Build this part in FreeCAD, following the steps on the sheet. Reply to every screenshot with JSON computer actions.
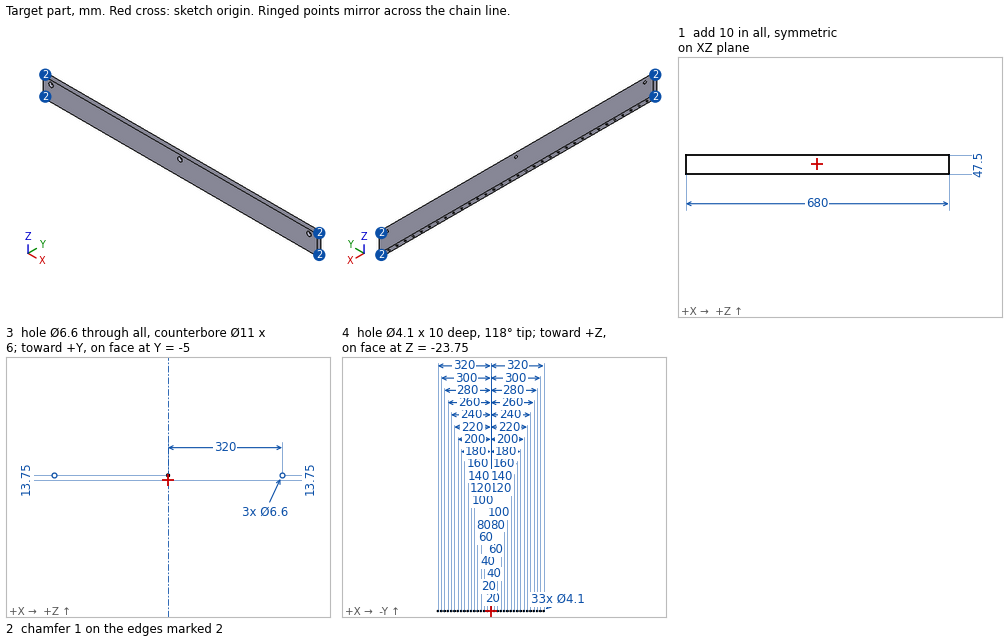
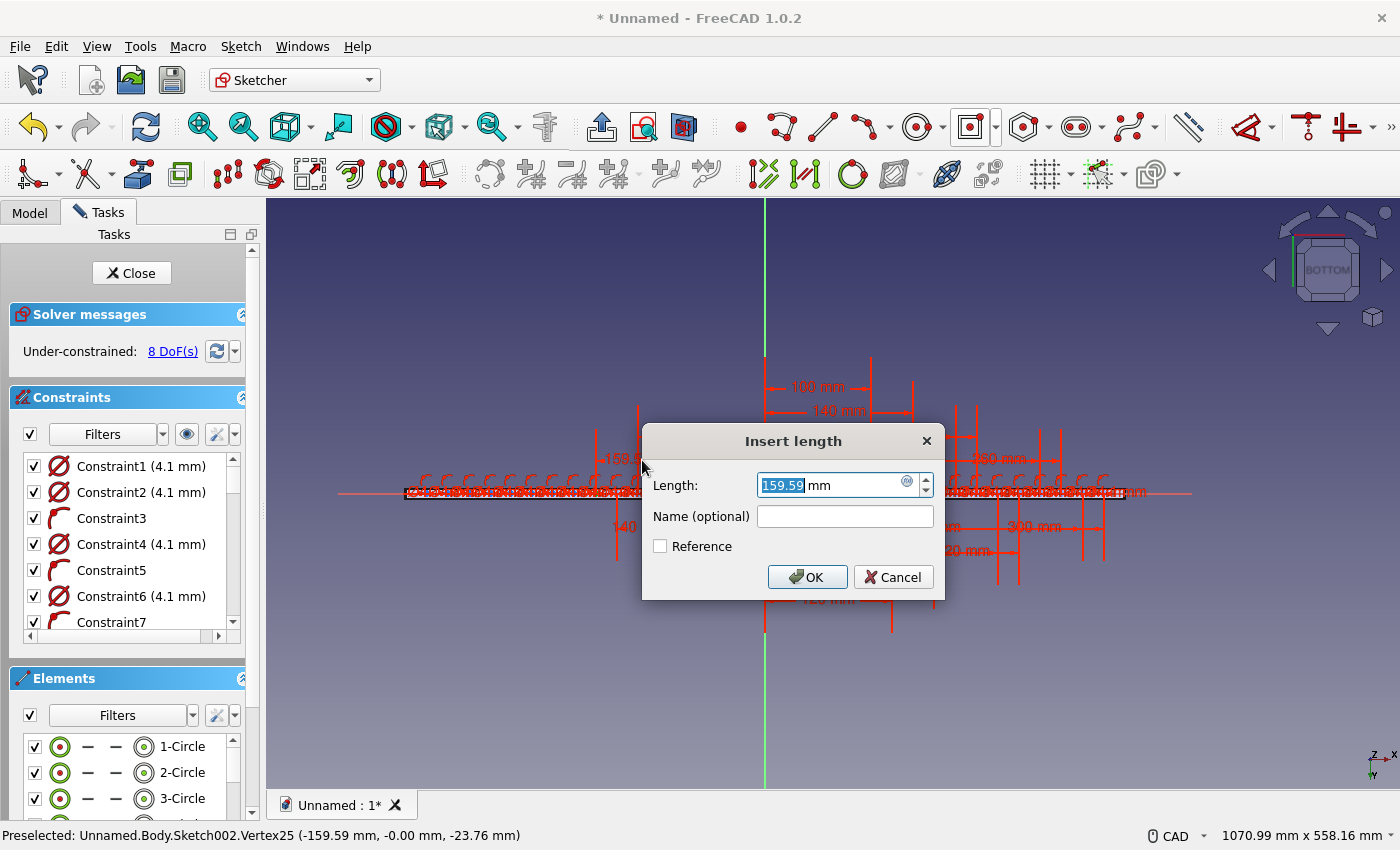
{"action": "type", "text": "160"}
{"action": "key", "text": "Return"}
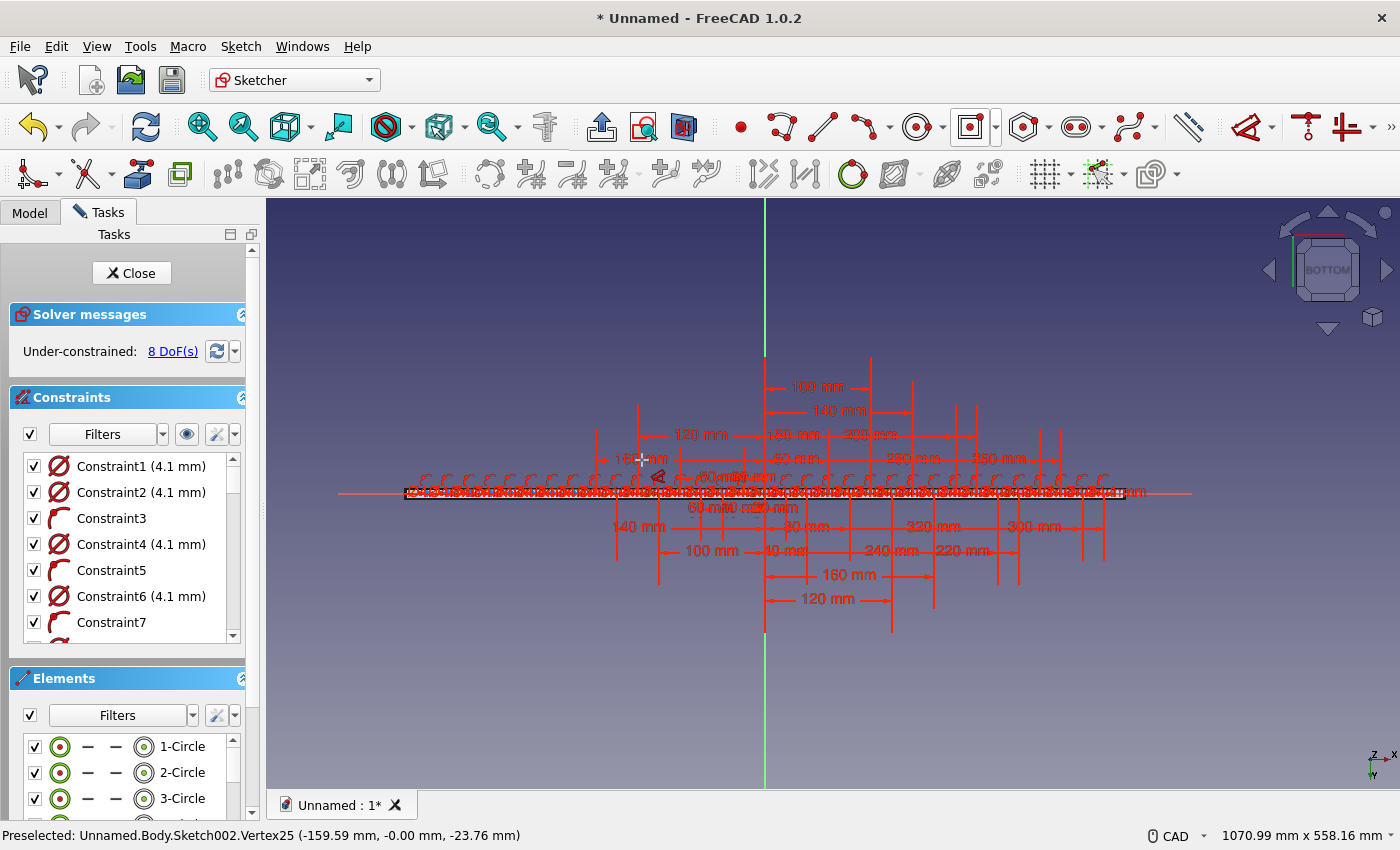
{"action": "left_click", "coordinate": [574, 494]}
{"action": "left_click", "coordinate": [626, 552]}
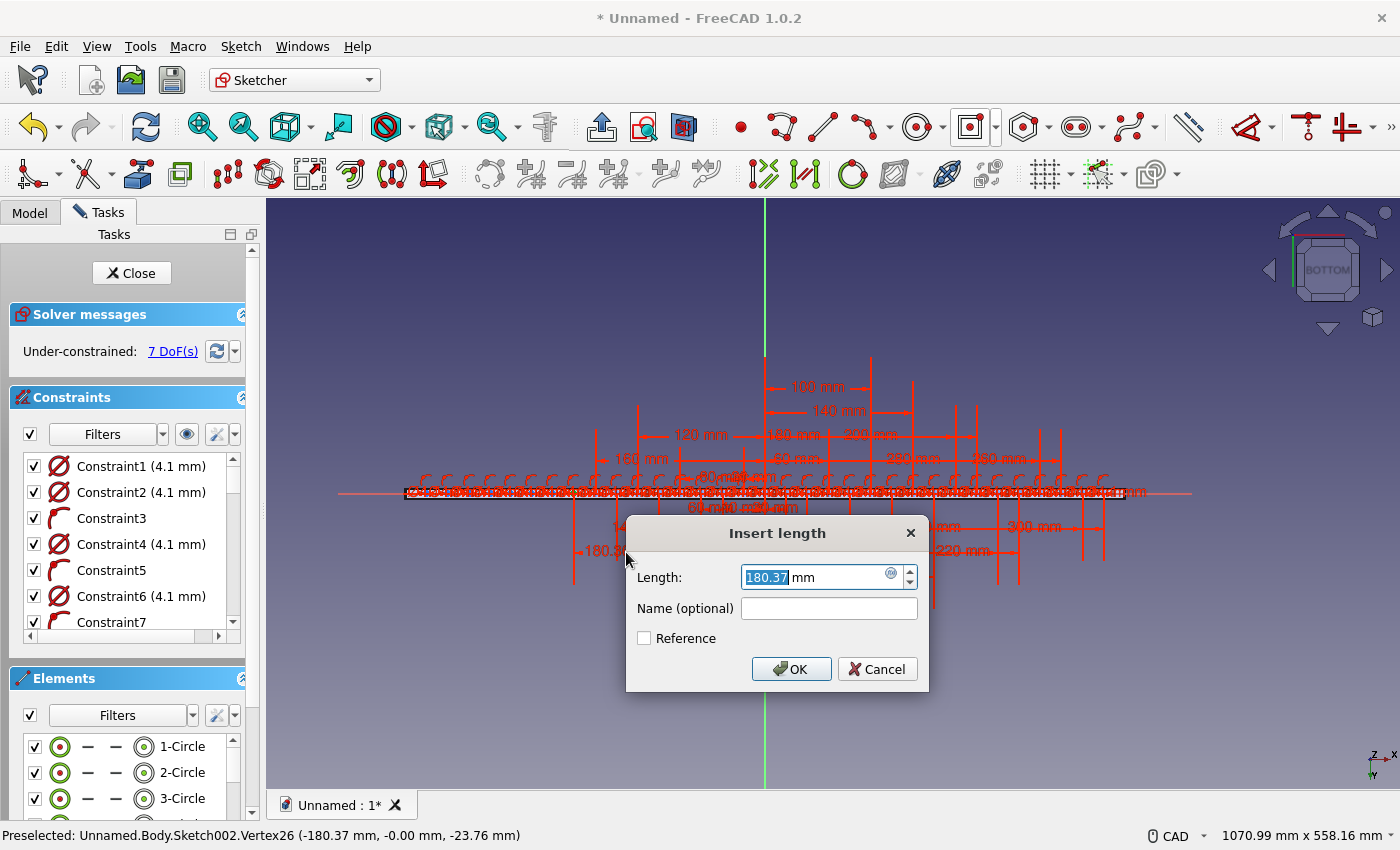
{"action": "type", "text": "180"}
{"action": "key", "text": "Return"}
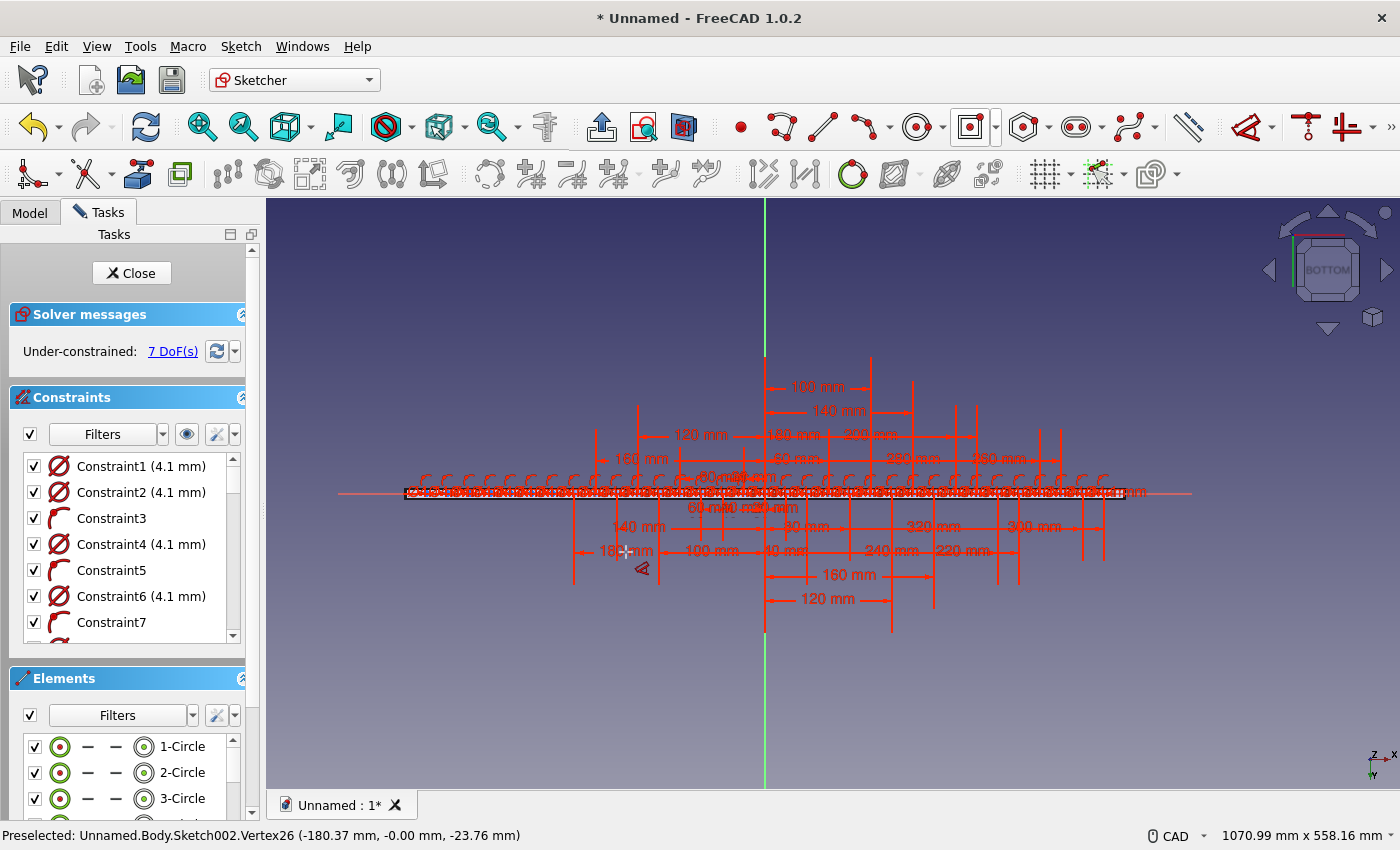
{"action": "left_click", "coordinate": [553, 494]}
{"action": "left_click", "coordinate": [610, 436]}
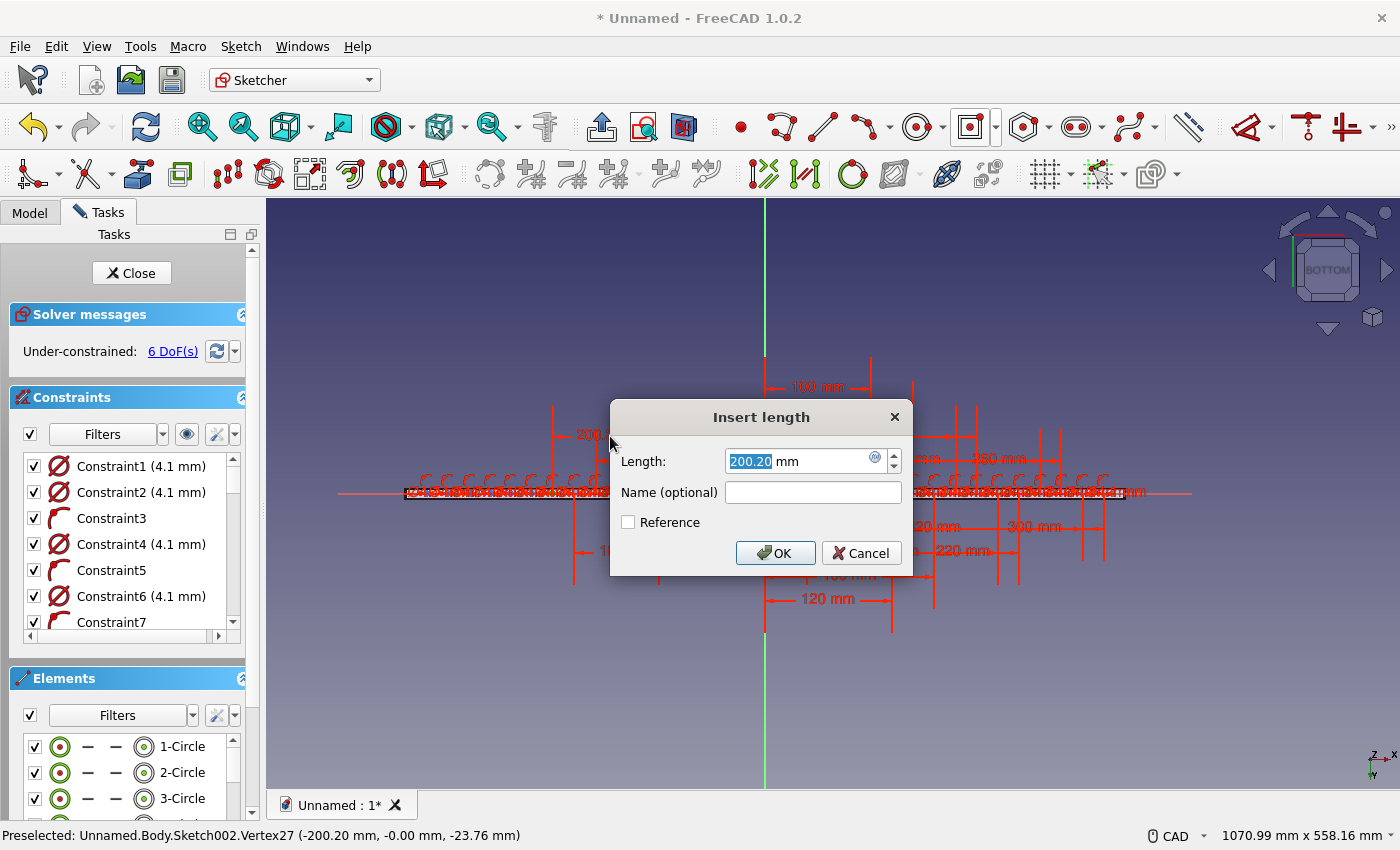
{"action": "type", "text": "200"}
{"action": "key", "text": "Return"}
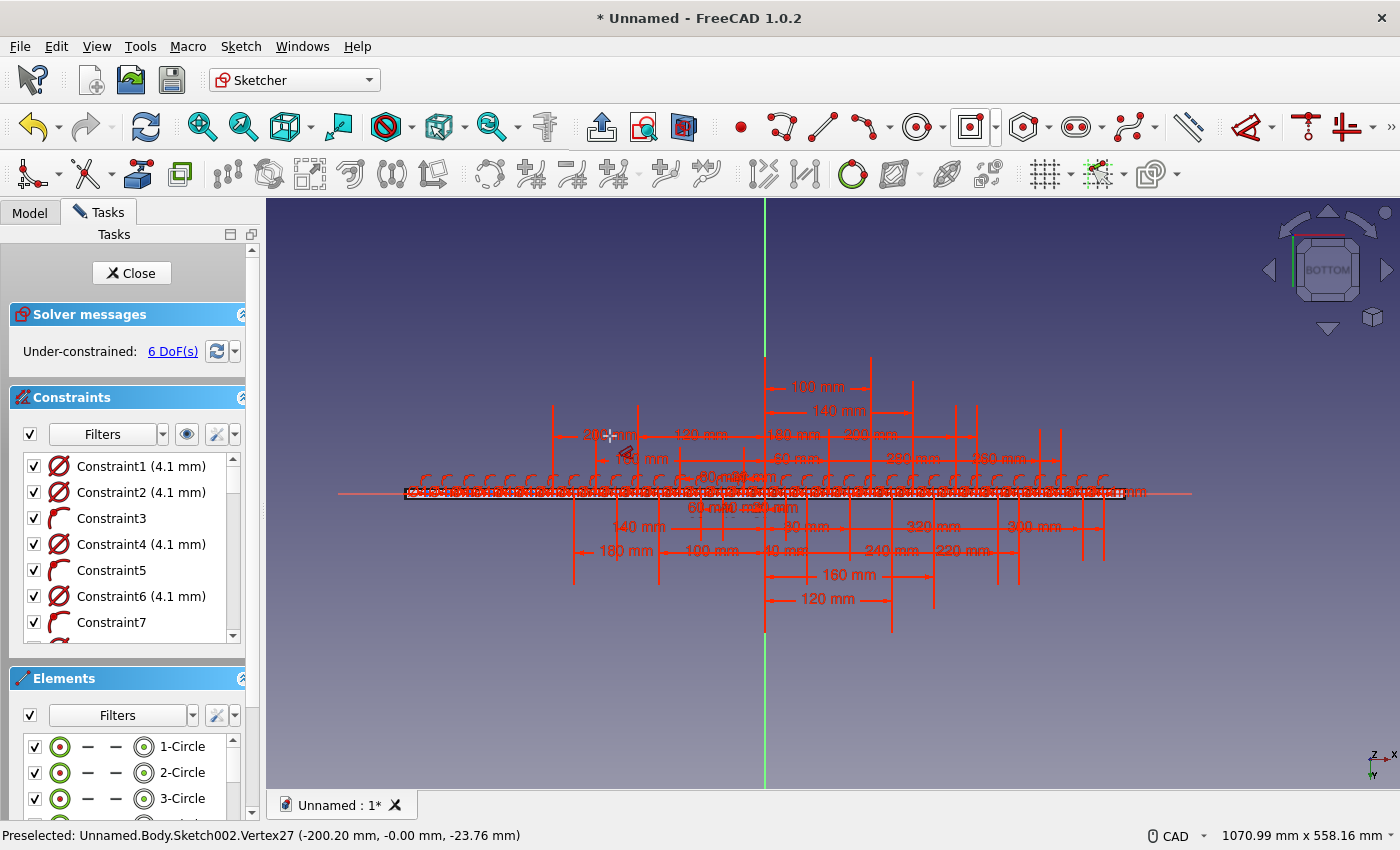
{"action": "left_click", "coordinate": [532, 494]}
{"action": "left_click", "coordinate": [567, 528]}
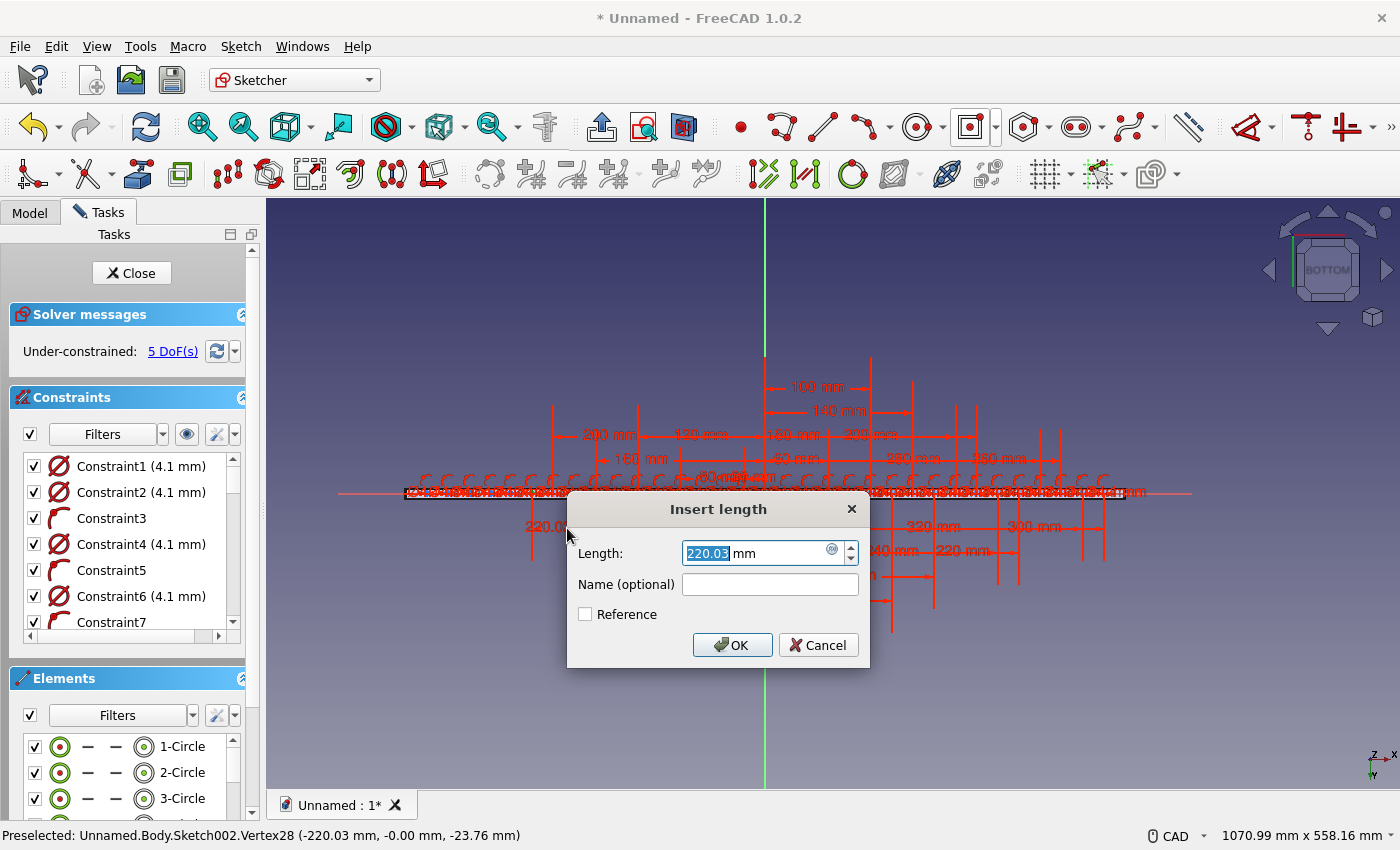
{"action": "type", "text": "220"}
{"action": "key", "text": "Return"}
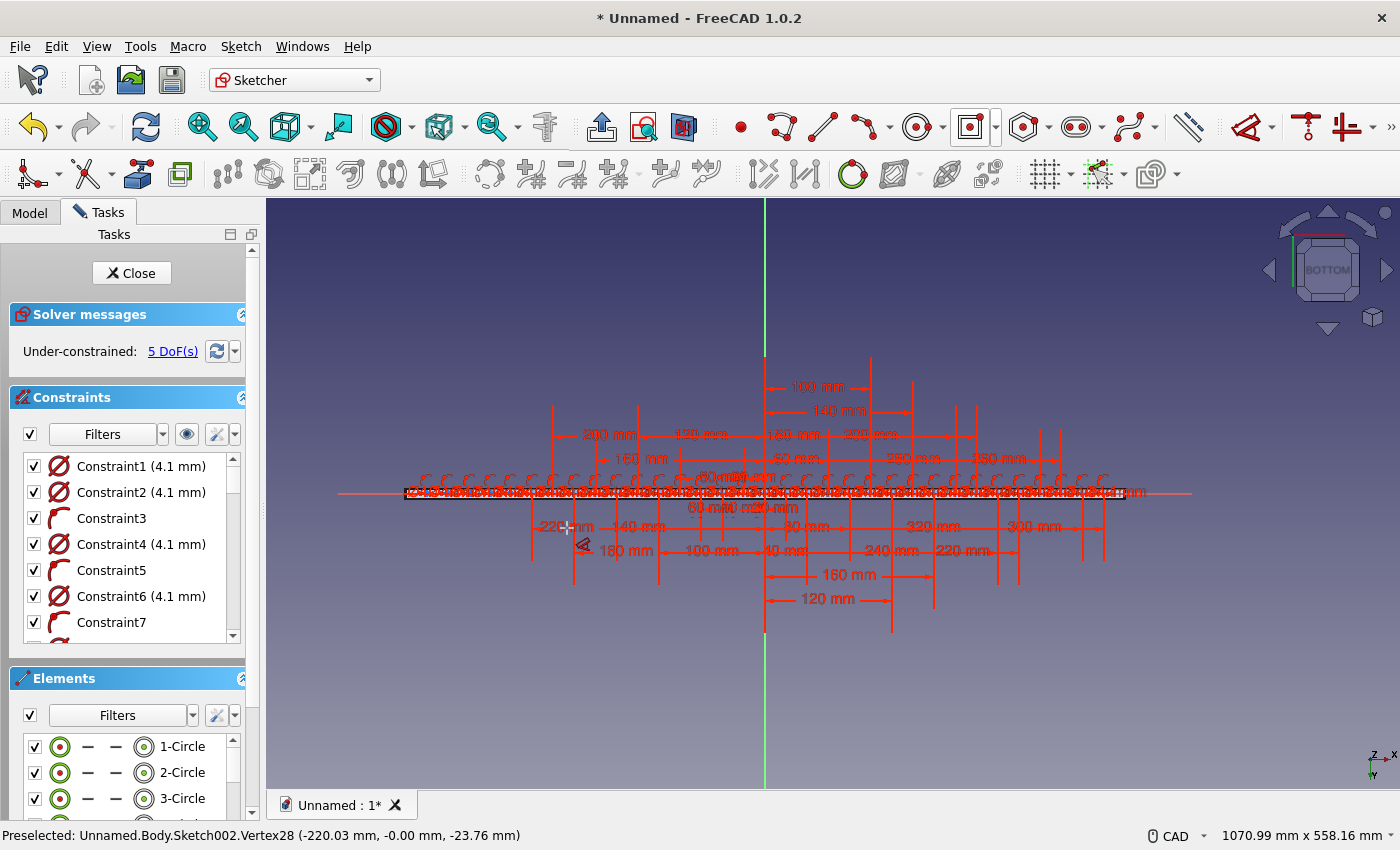
{"action": "left_click", "coordinate": [511, 494]}
{"action": "left_click", "coordinate": [549, 460]}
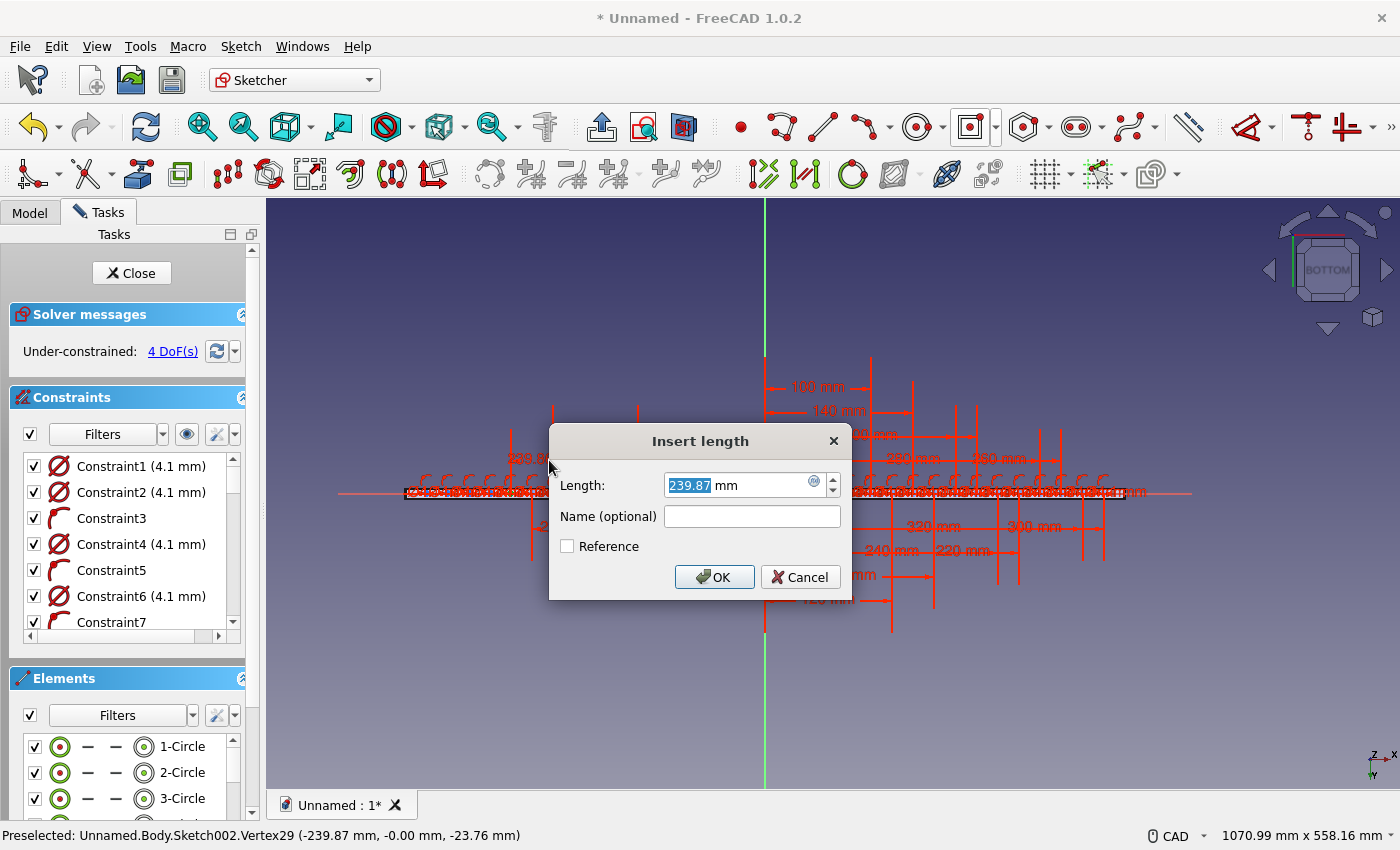
{"action": "type", "text": "240"}
{"action": "key", "text": "Return"}